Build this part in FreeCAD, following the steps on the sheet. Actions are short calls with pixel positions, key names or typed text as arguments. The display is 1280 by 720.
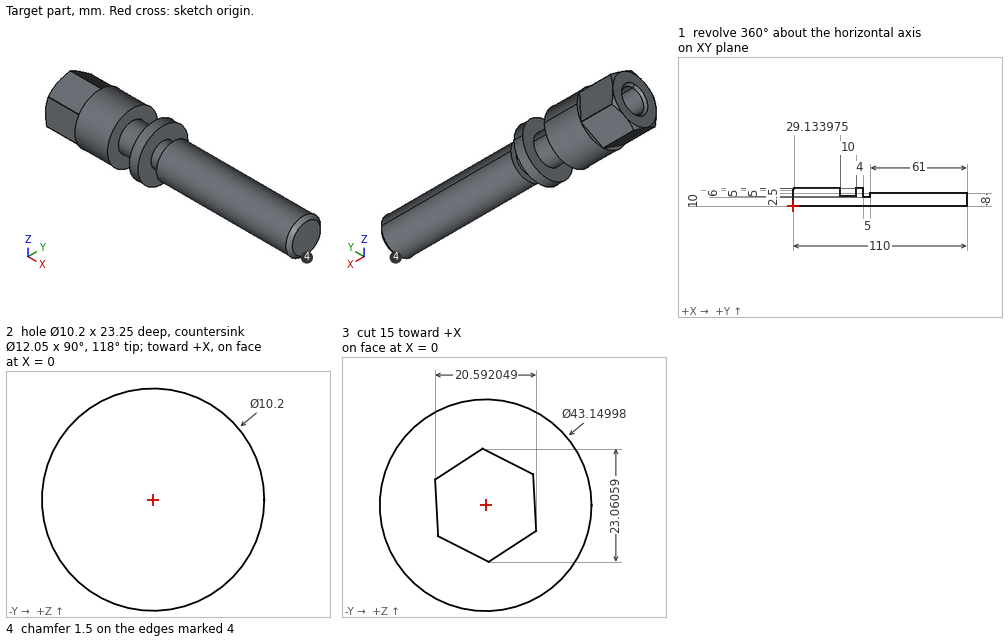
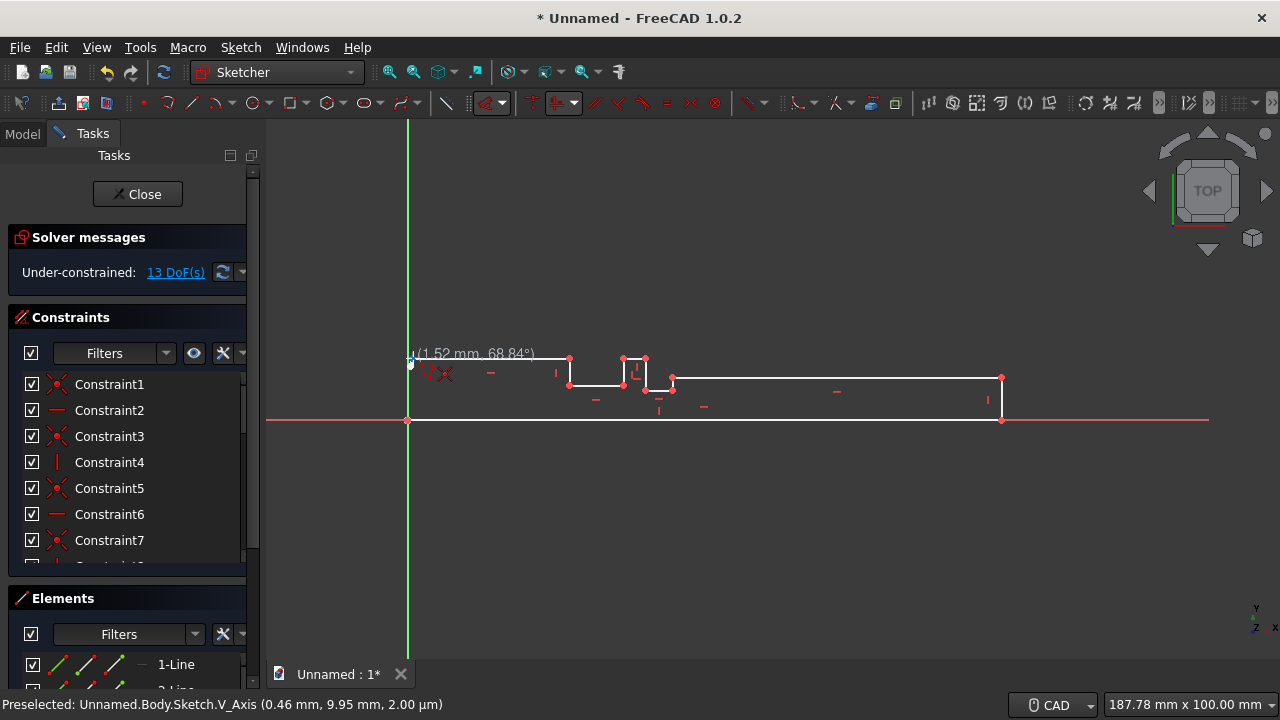
click(408, 420)
key(Escape)
key(Escape)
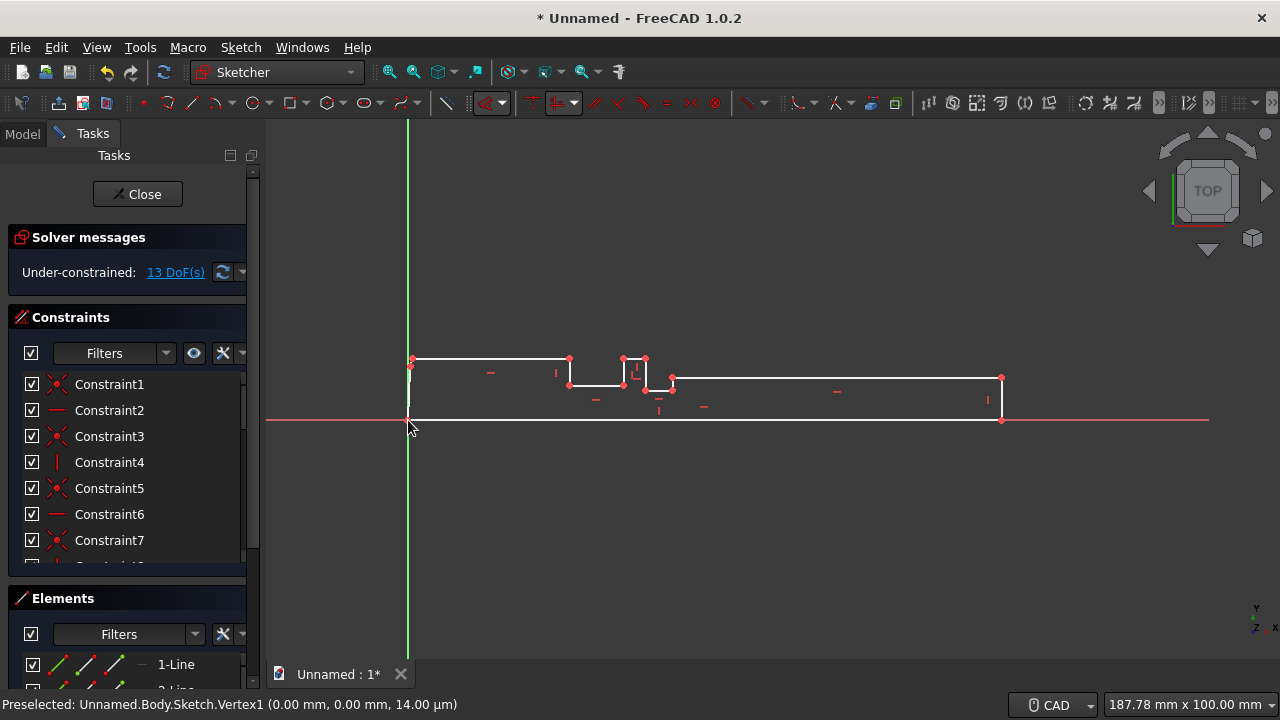
click(409, 382)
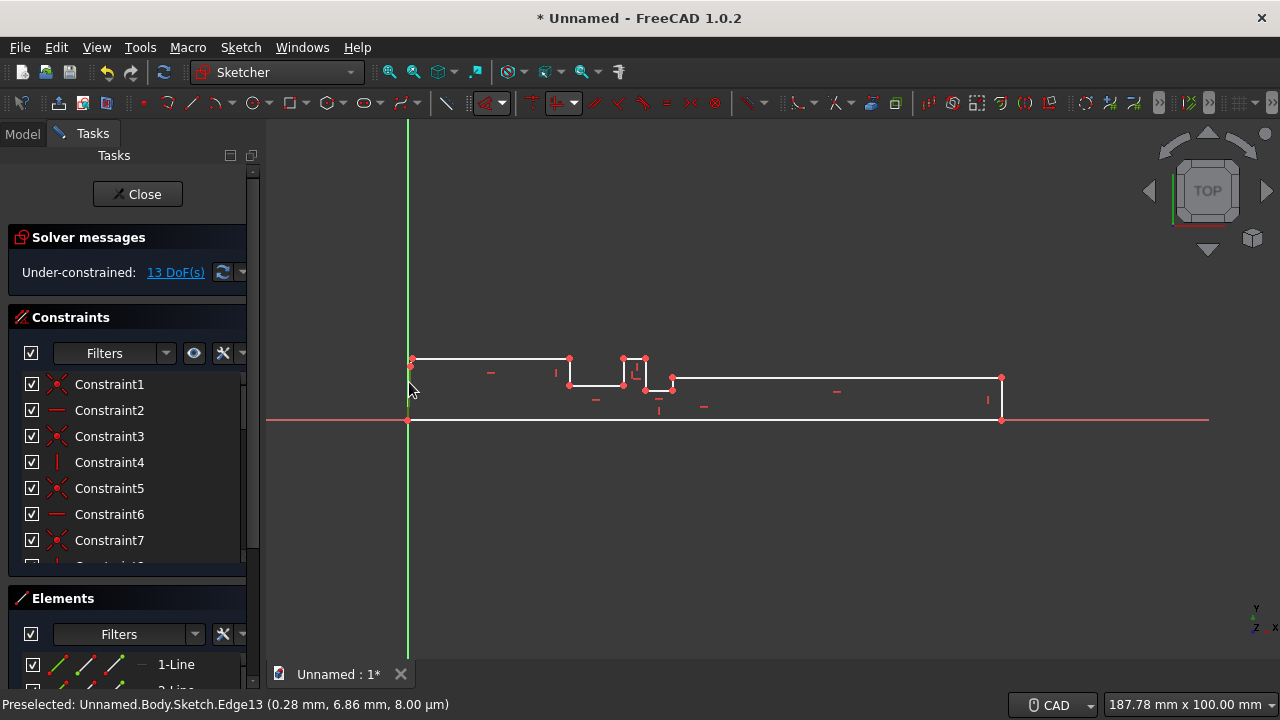
click(576, 104)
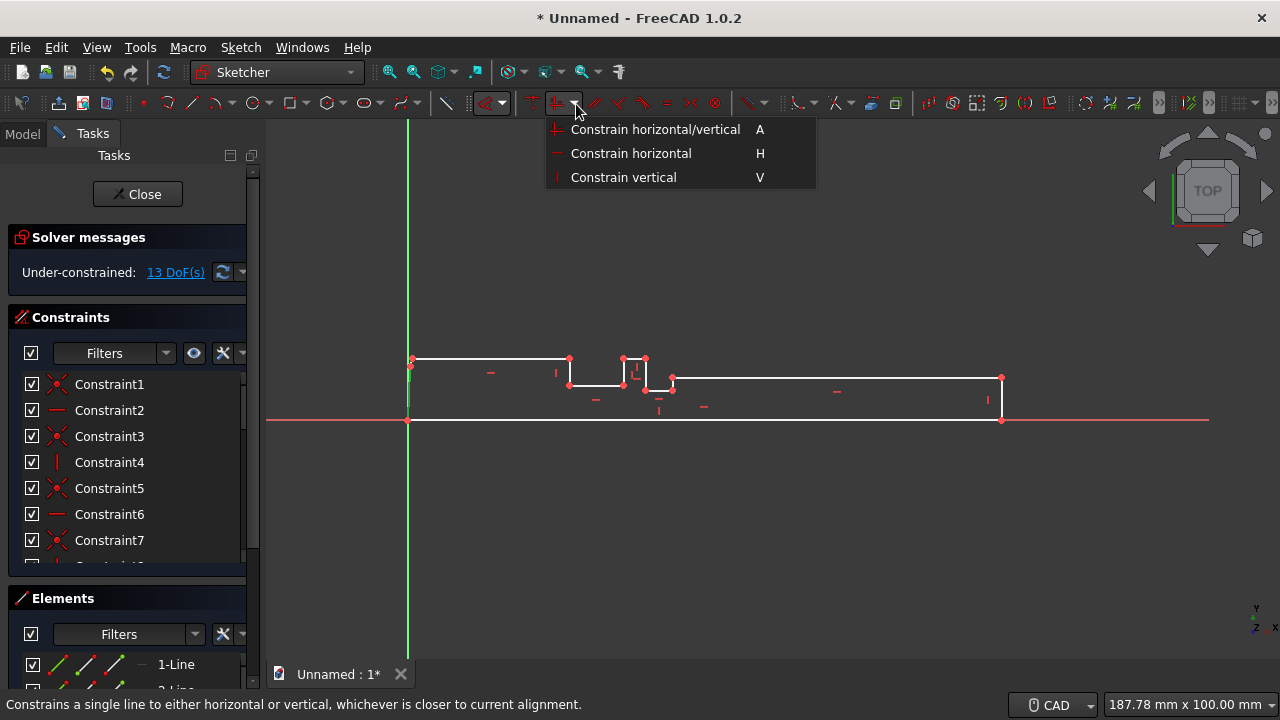
click(681, 177)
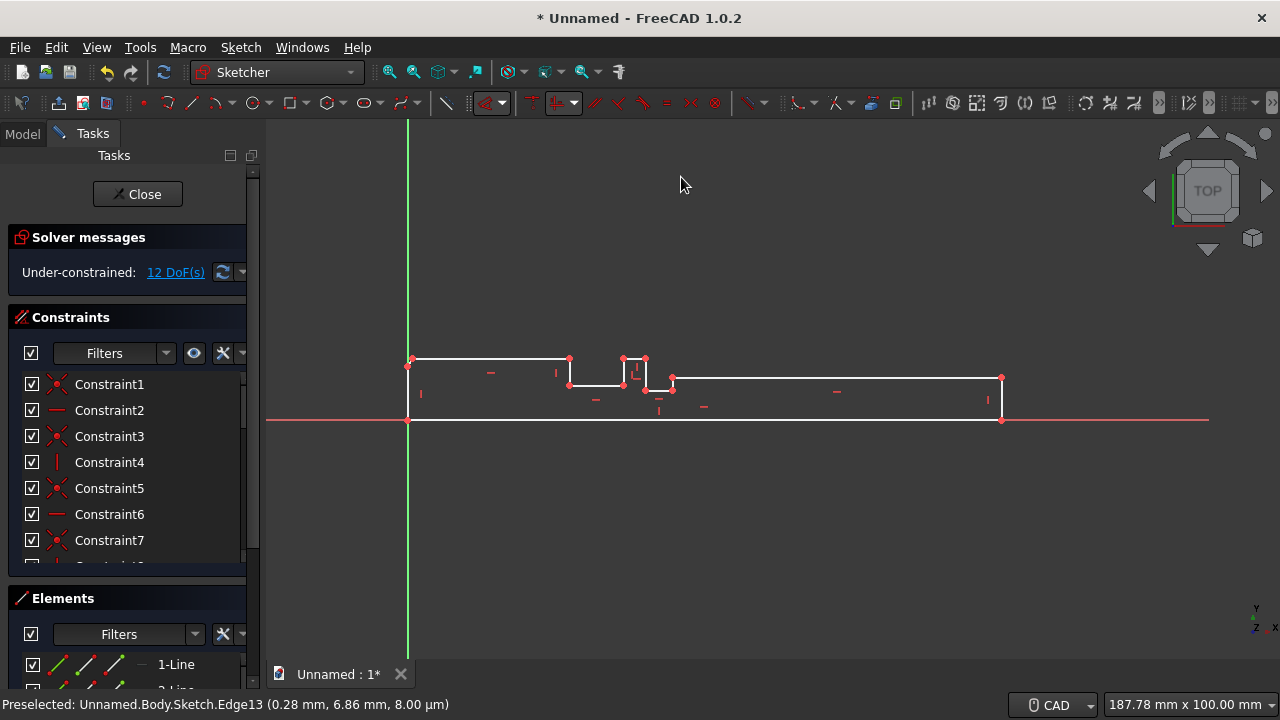
key(d)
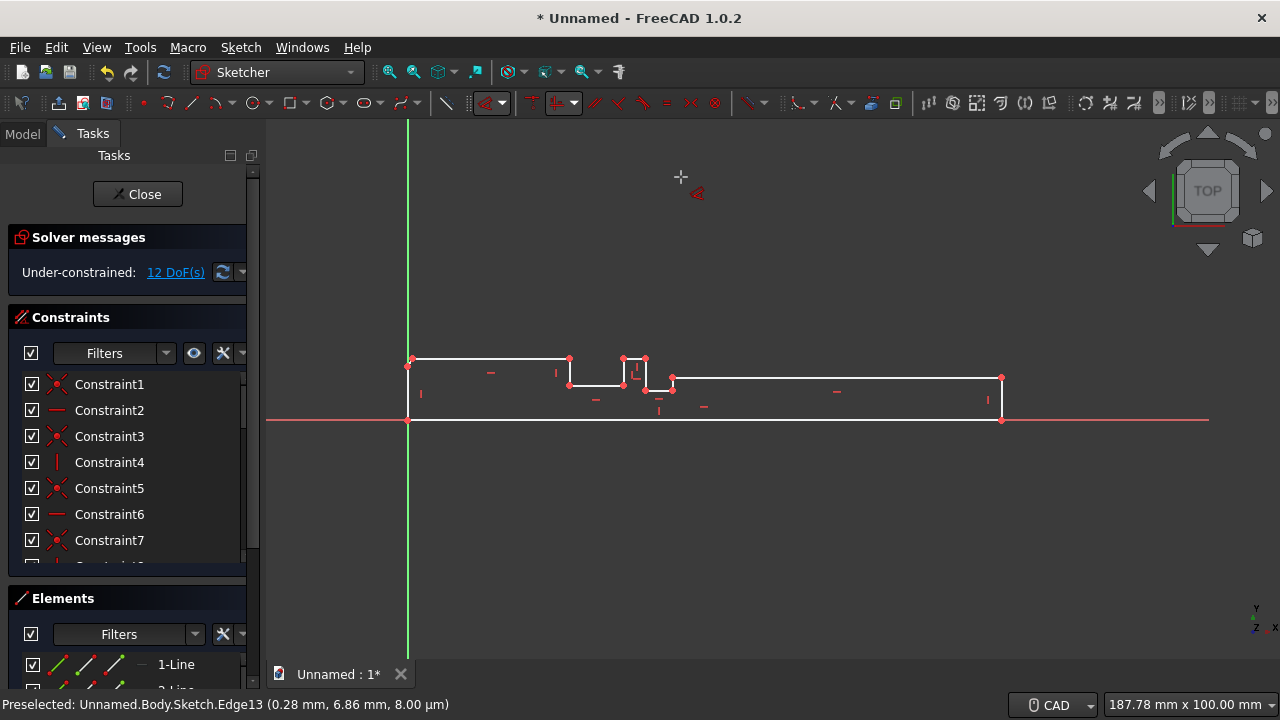
click(1002, 407)
click(1036, 399)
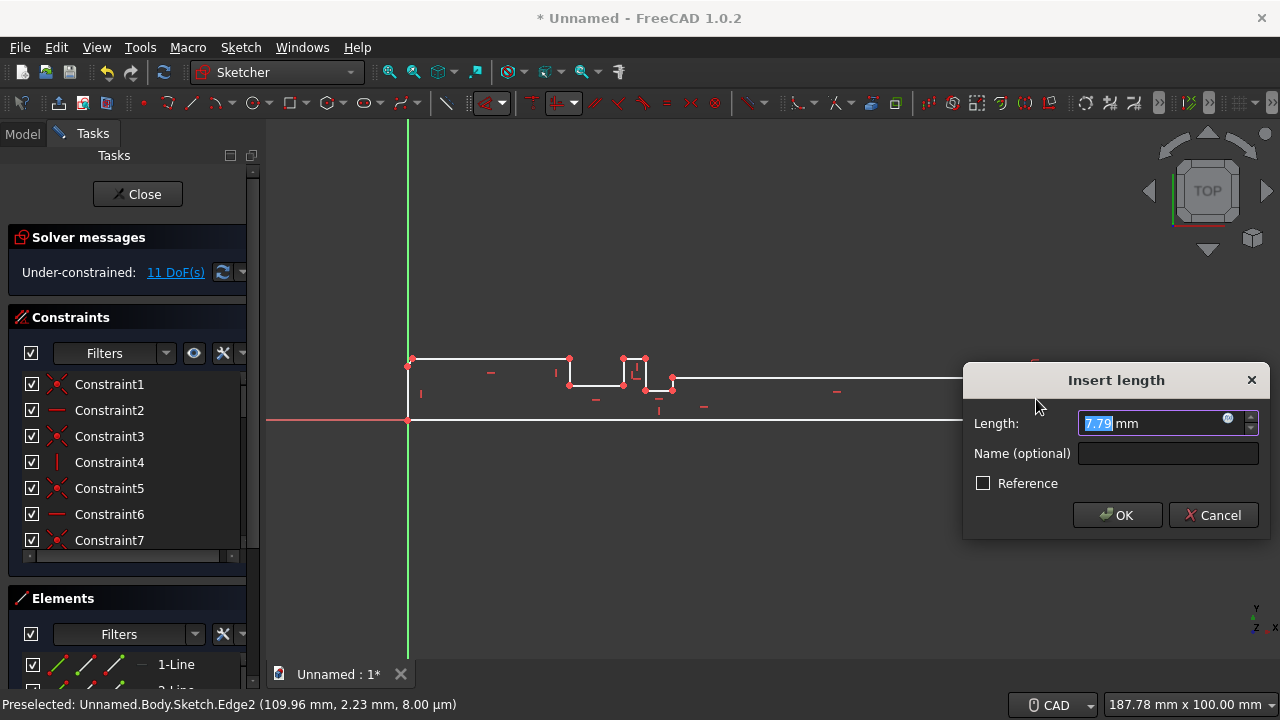
text(8)
key(Return)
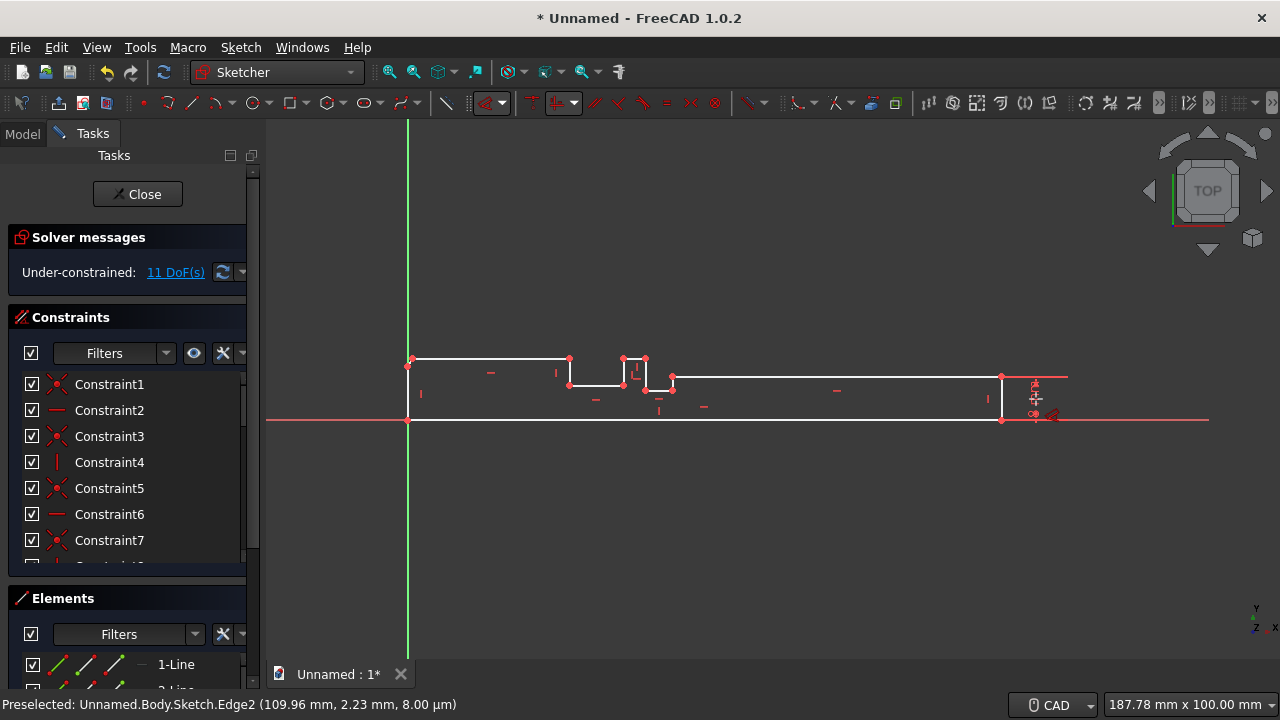
scroll(662, 391, up, 2)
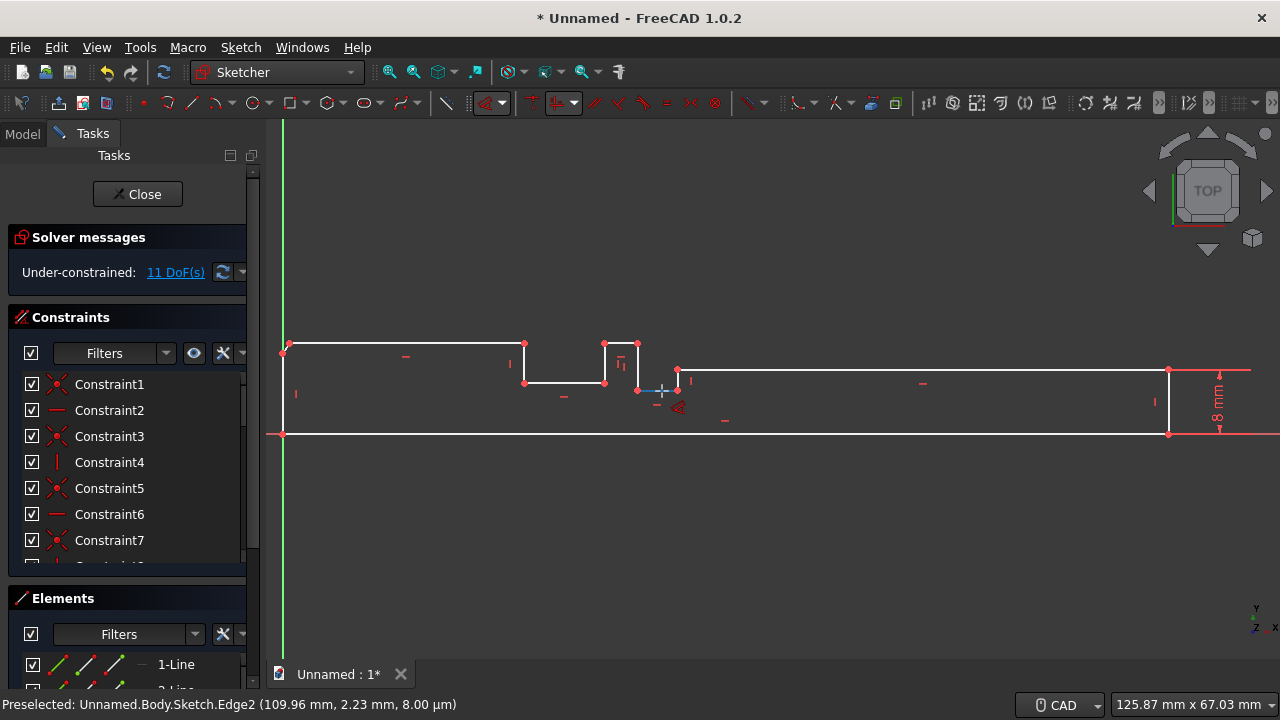
click(662, 391)
click(658, 357)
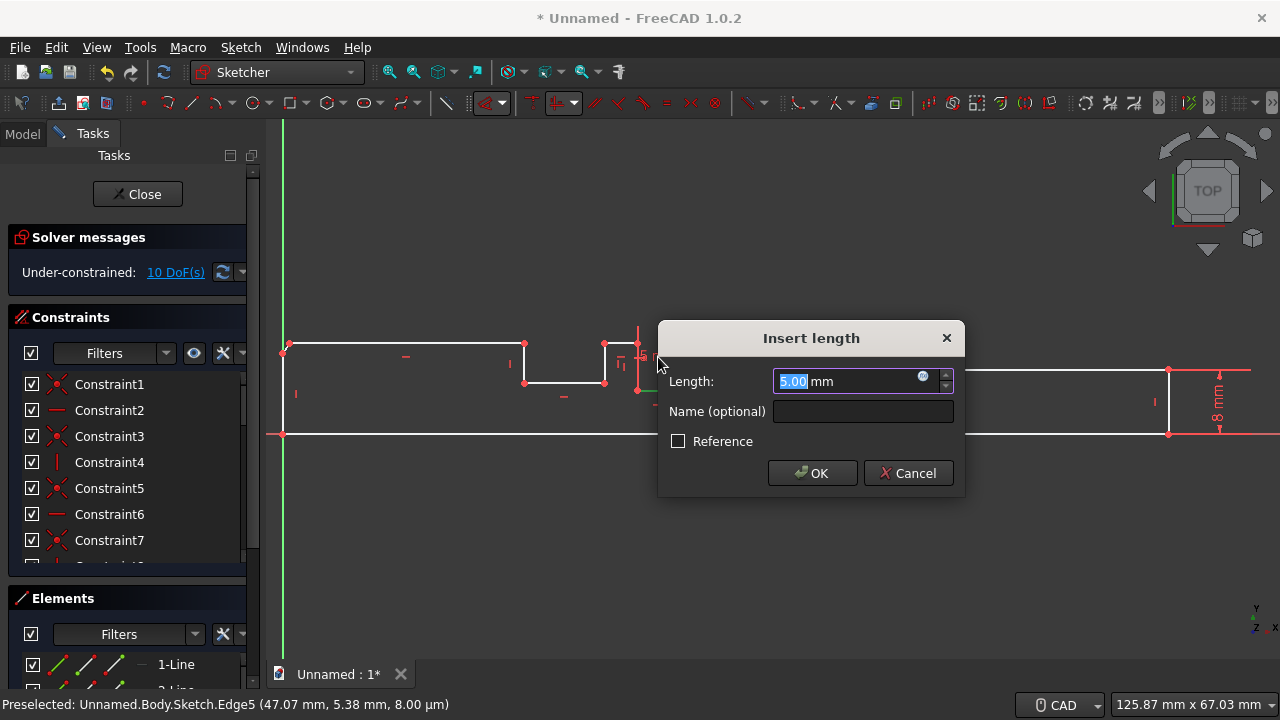
text(5)
key(Return)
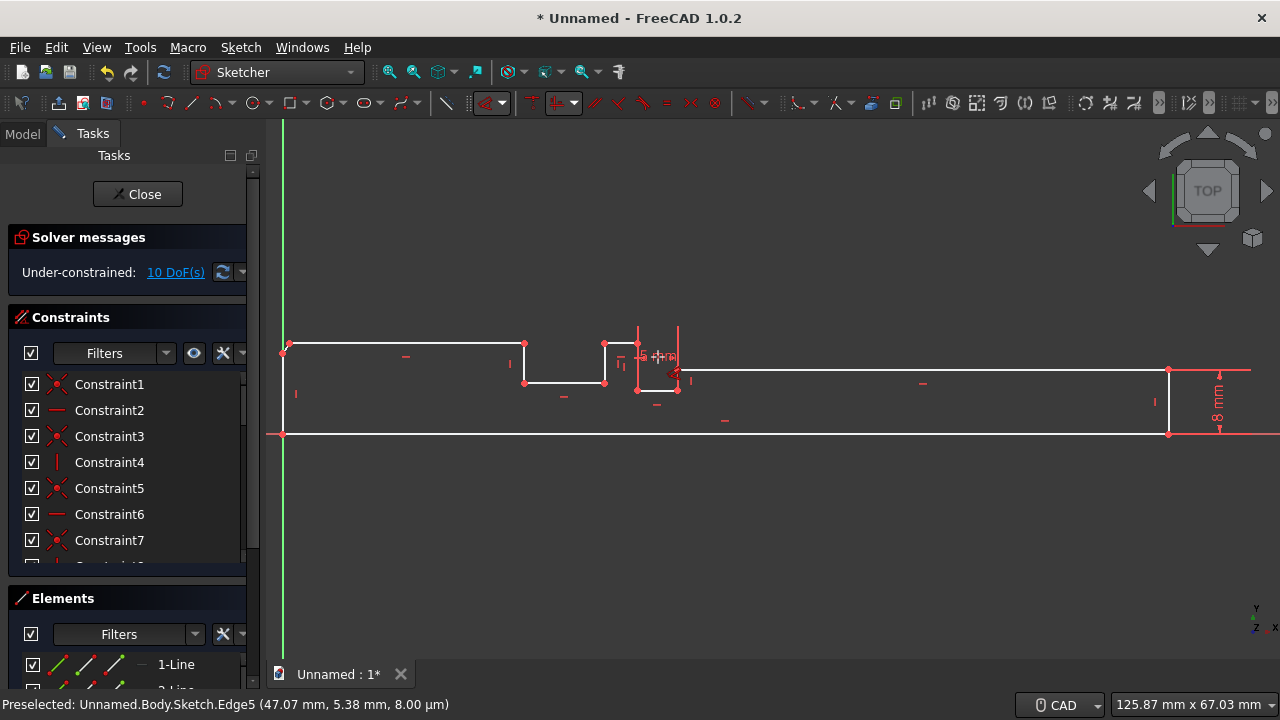
click(638, 376)
click(580, 367)